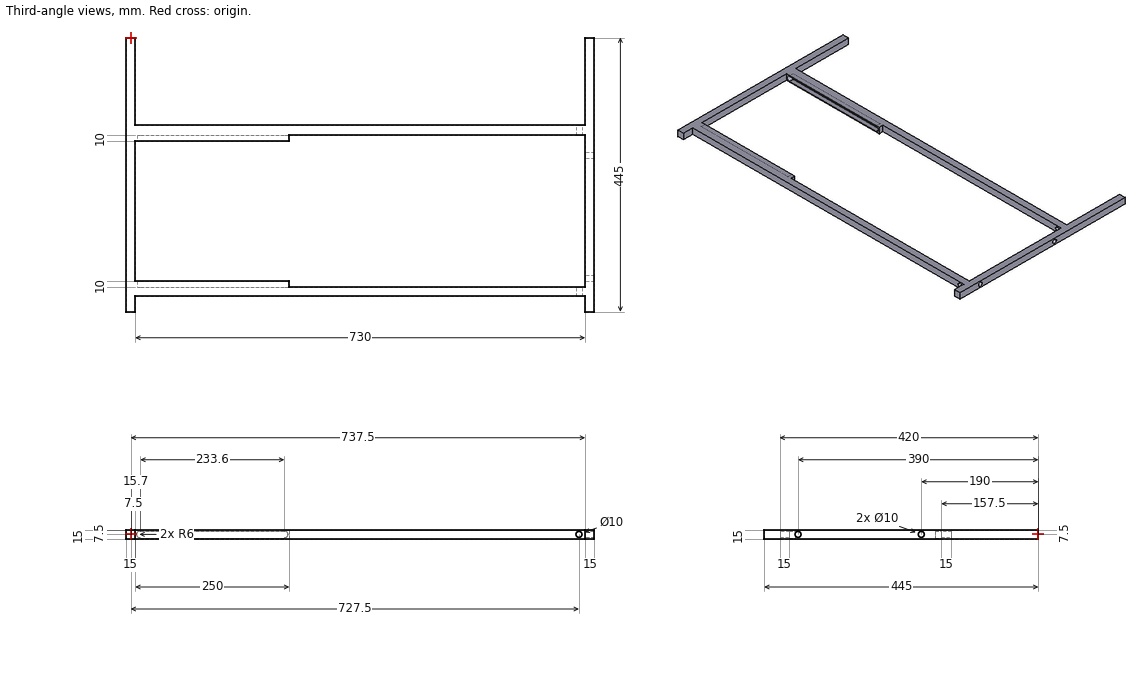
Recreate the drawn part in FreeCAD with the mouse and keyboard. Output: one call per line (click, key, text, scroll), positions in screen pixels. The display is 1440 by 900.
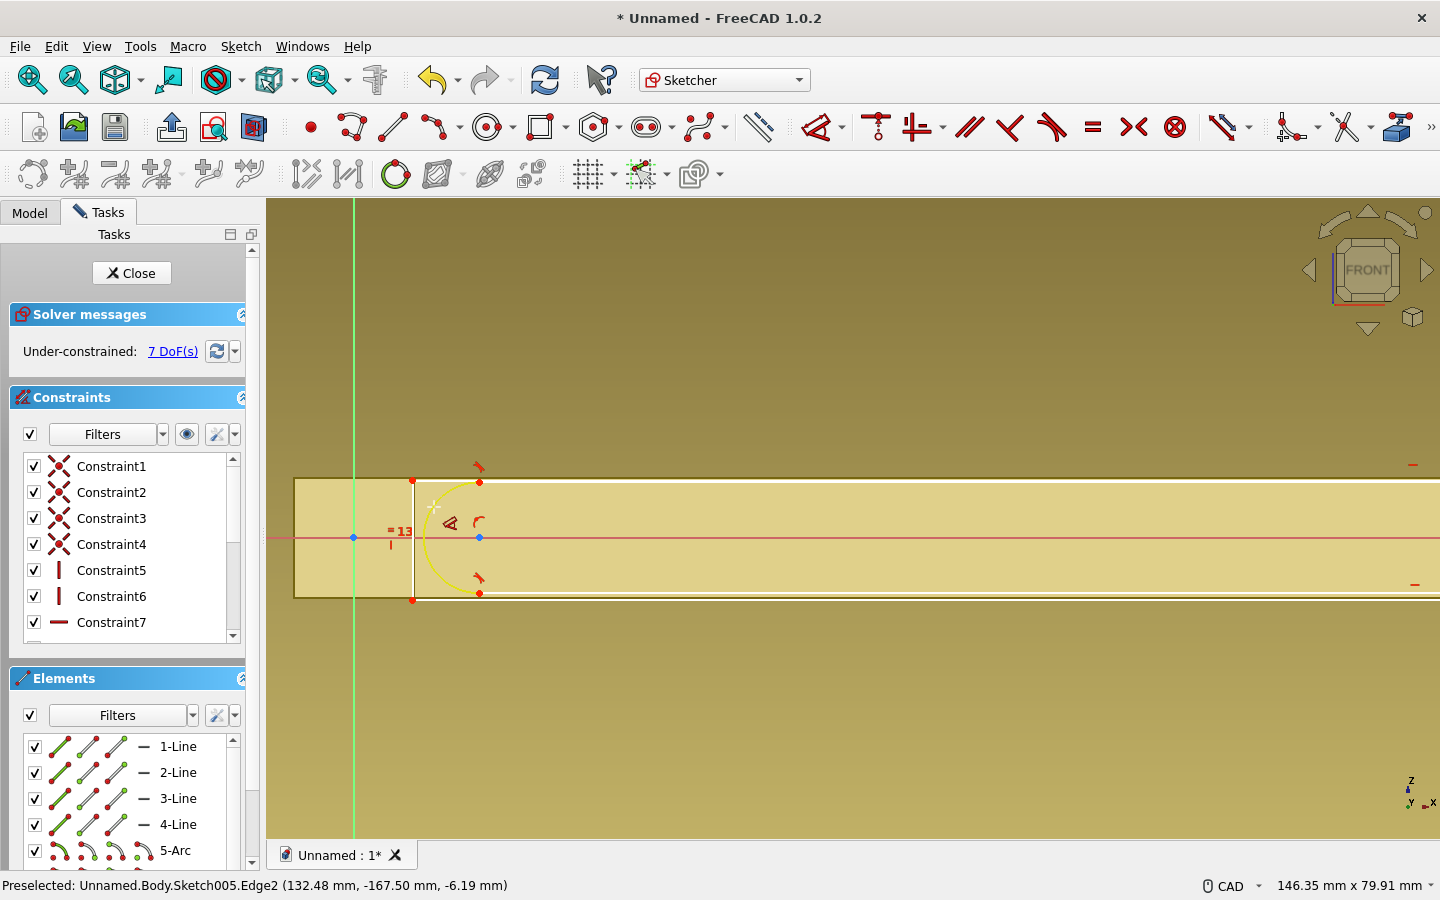
click(434, 505)
click(442, 458)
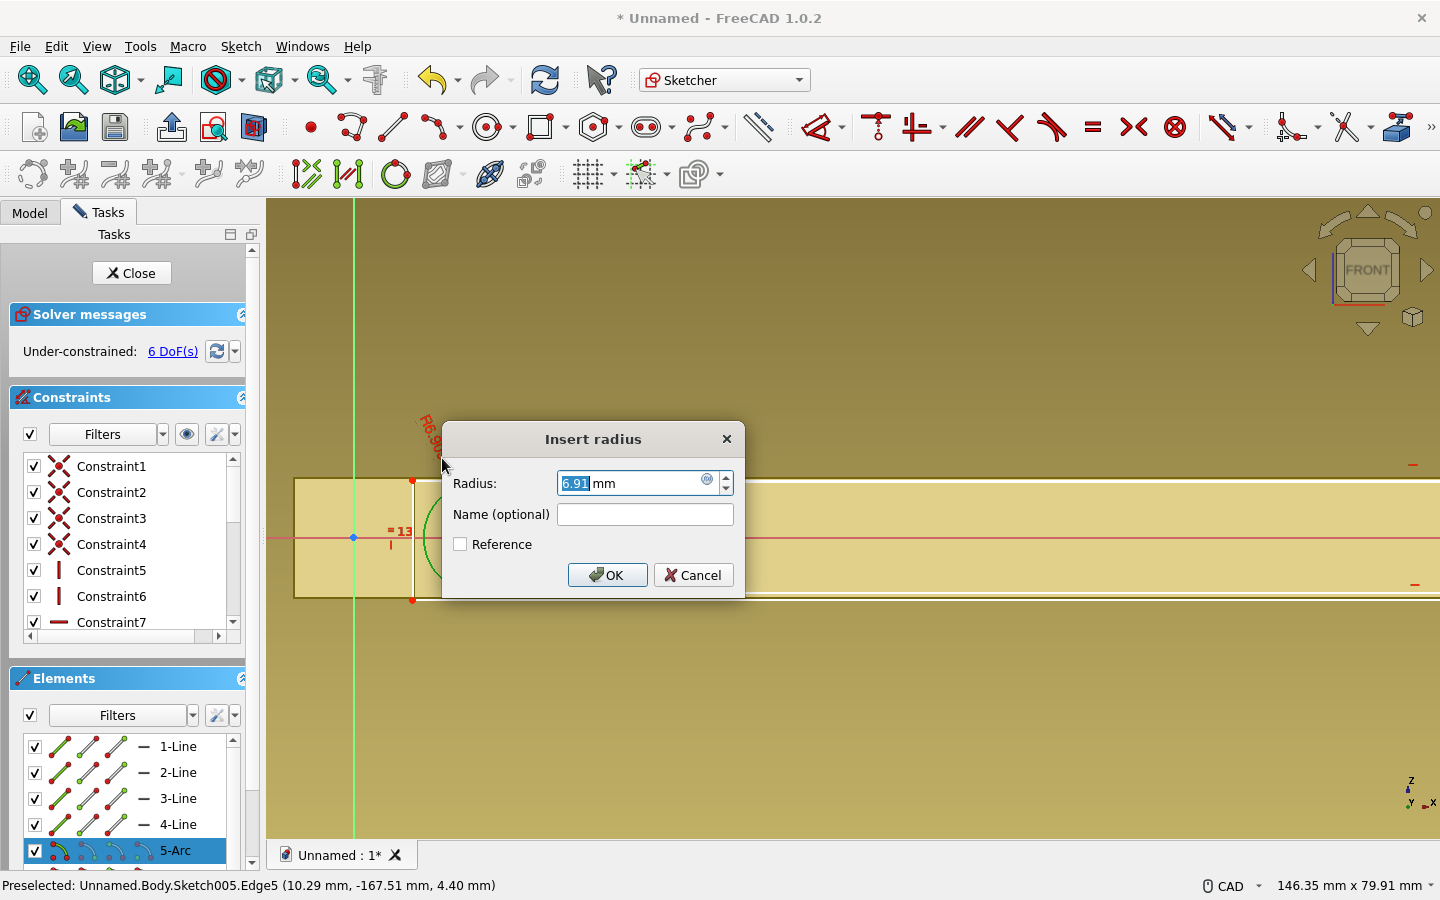
text(6)
key(Return)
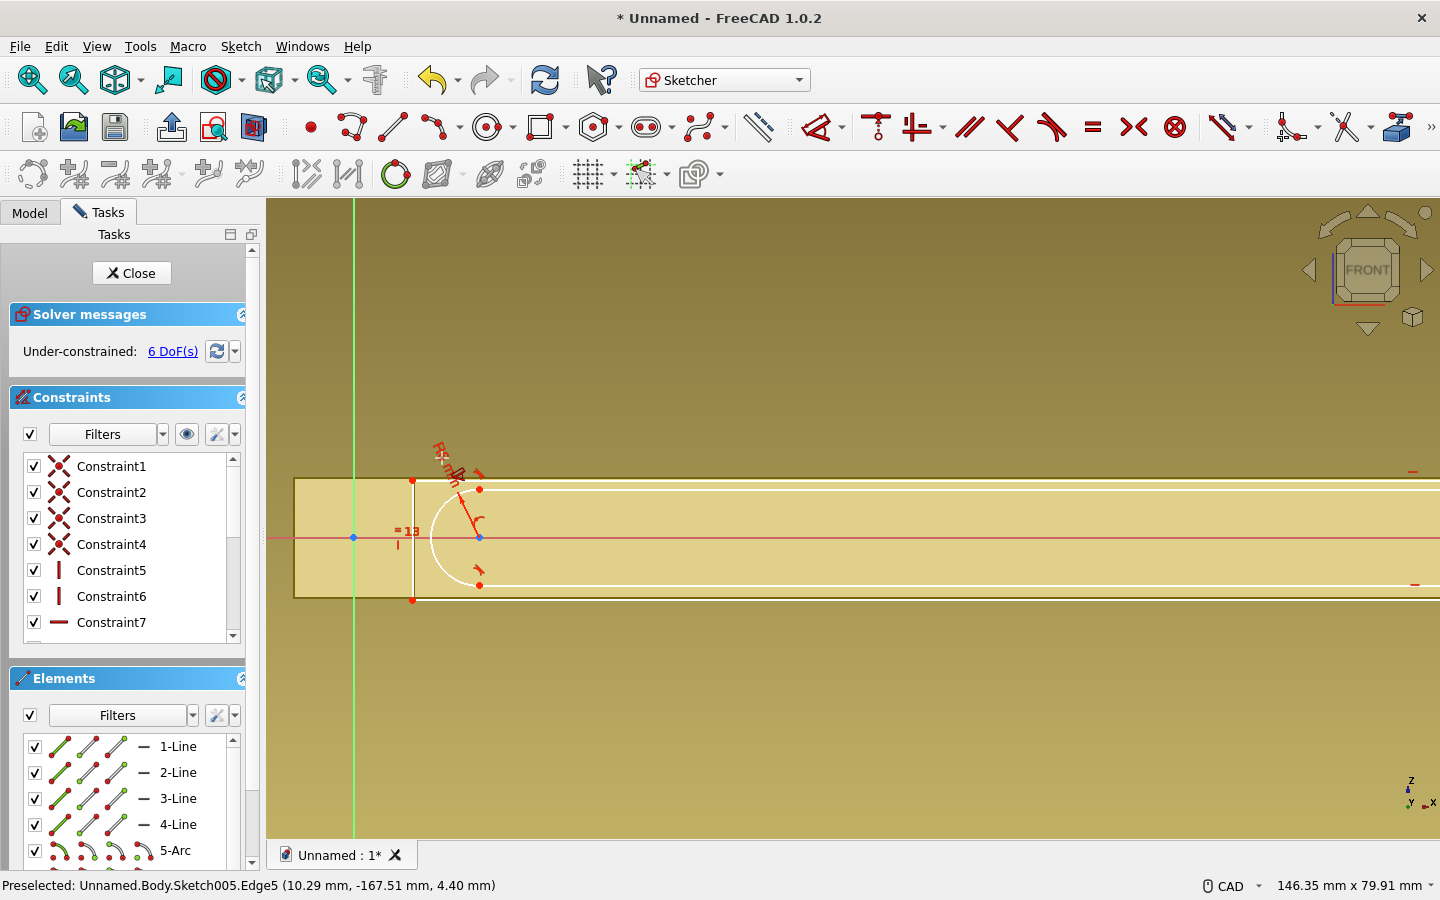
click(413, 517)
click(379, 513)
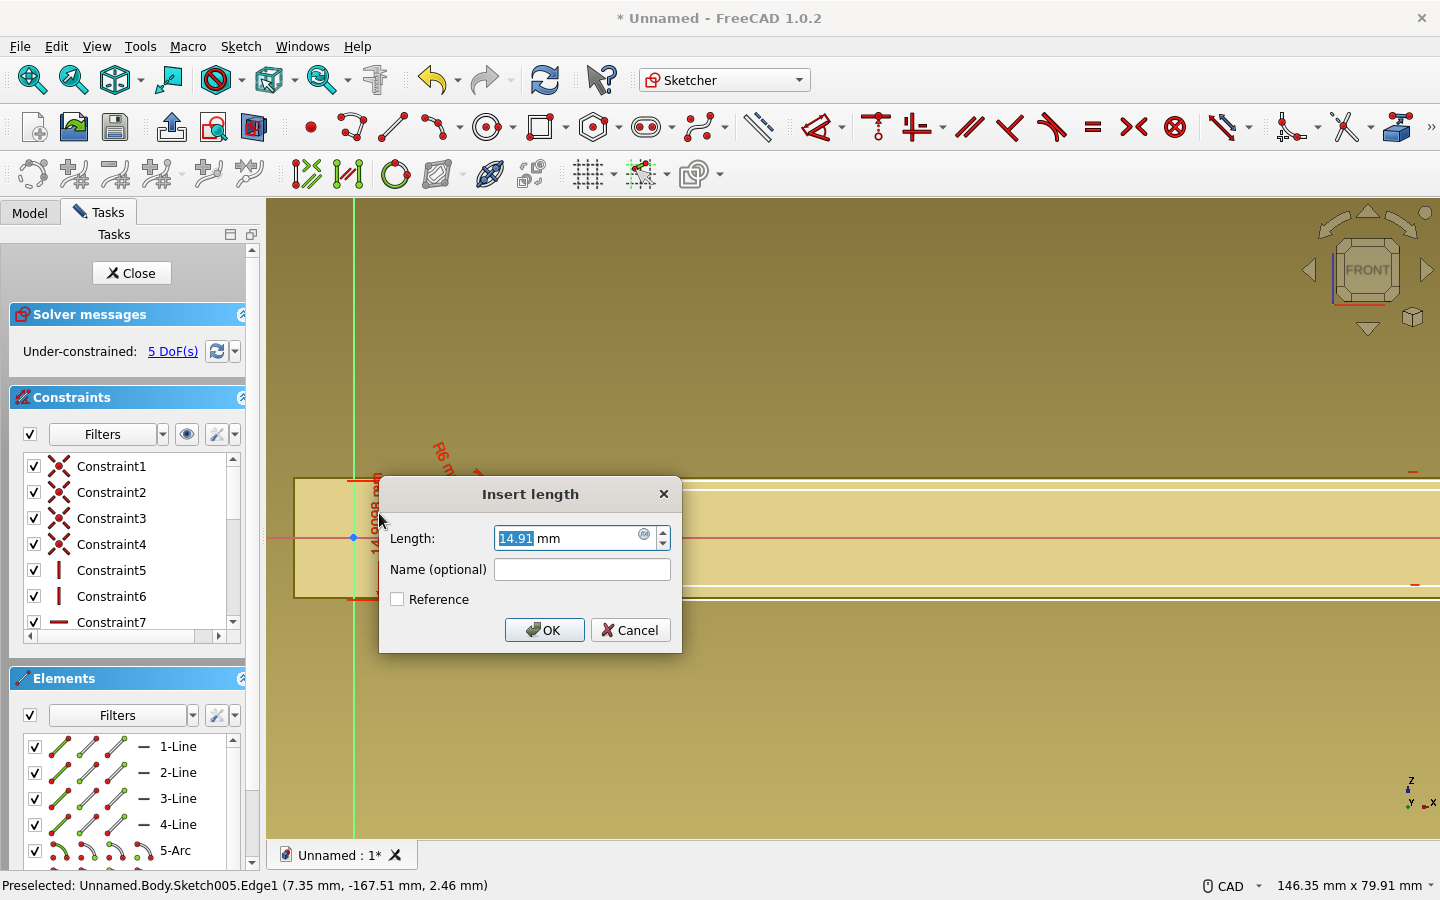
text(15)
key(Return)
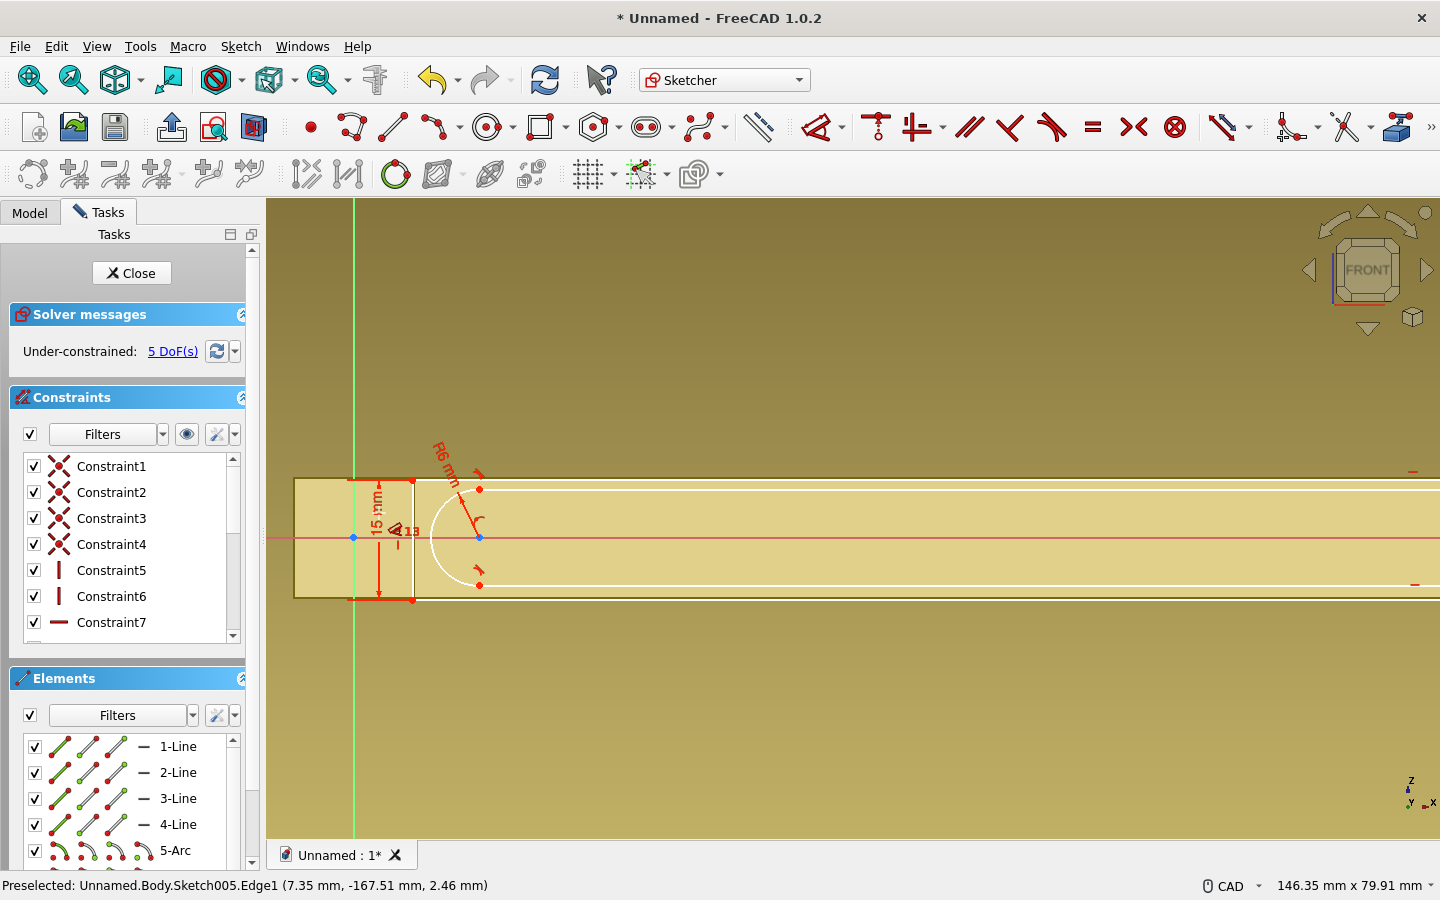
click(1015, 600)
click(844, 634)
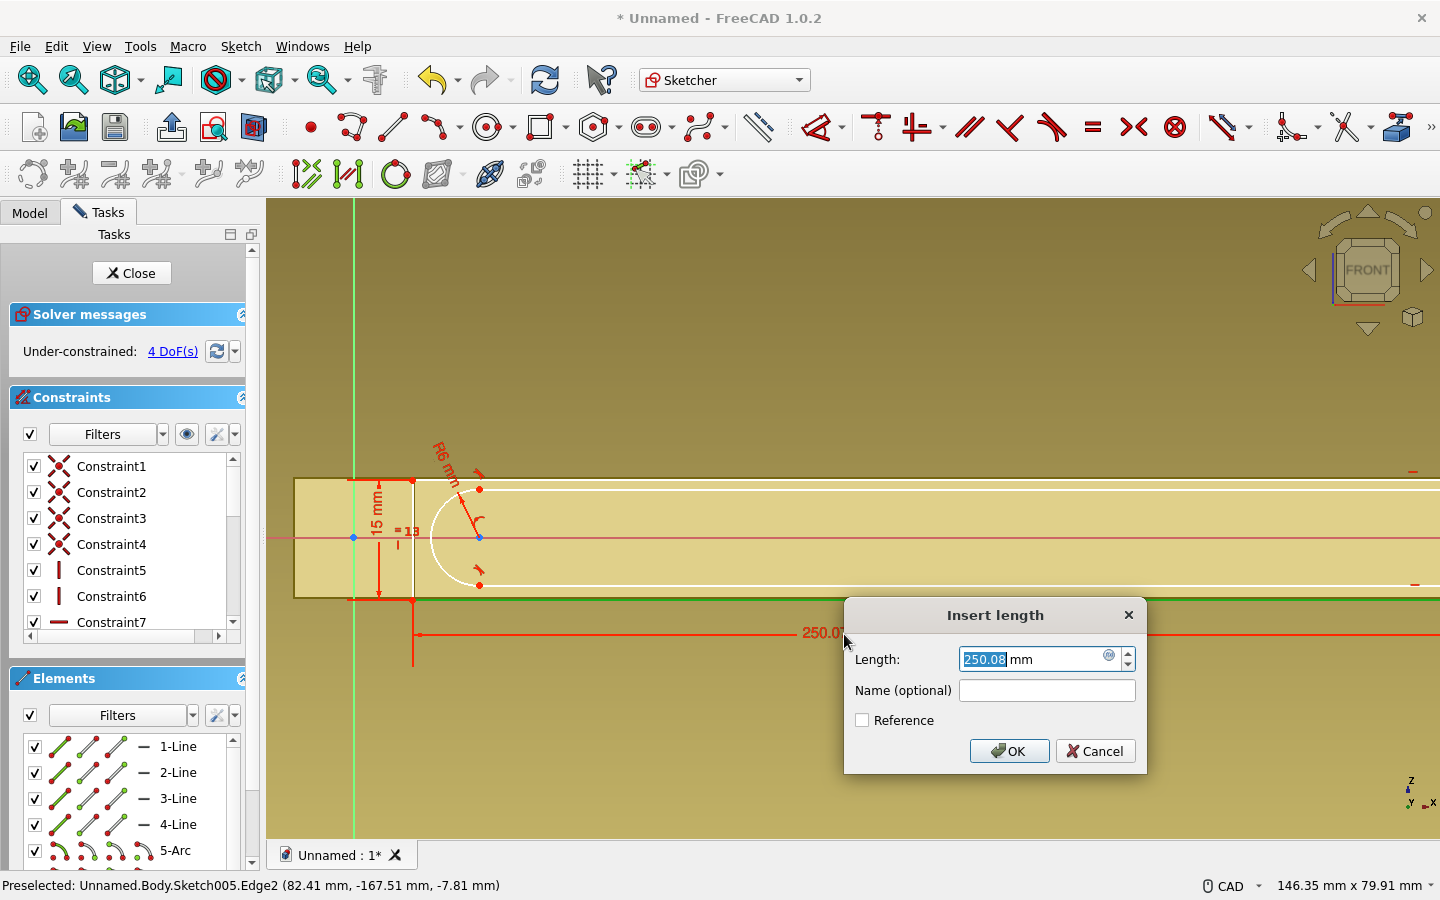
text(250)
key(Return)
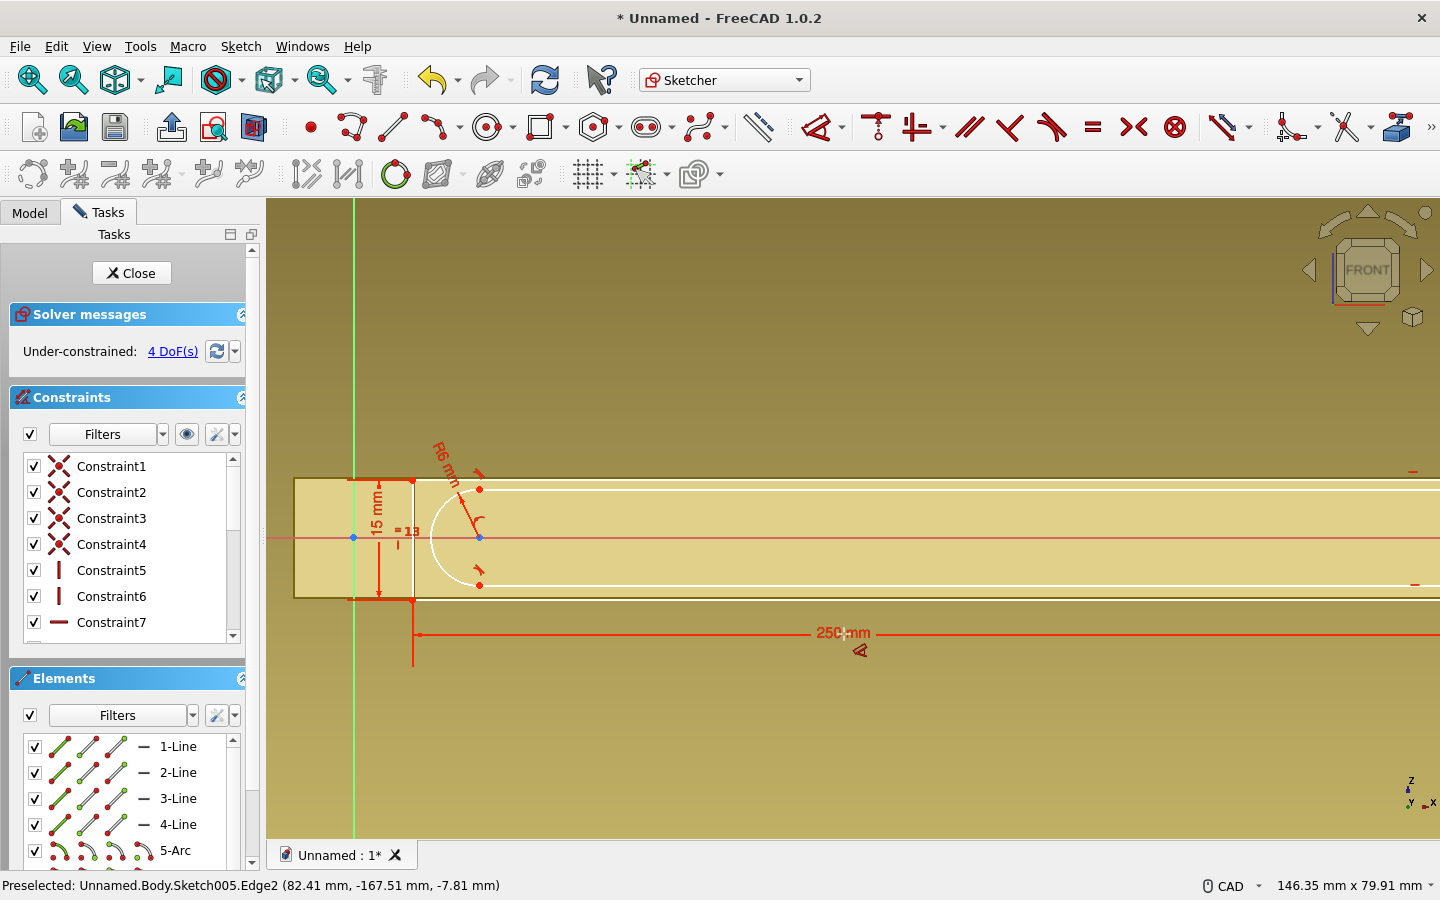
click(413, 480)
click(370, 446)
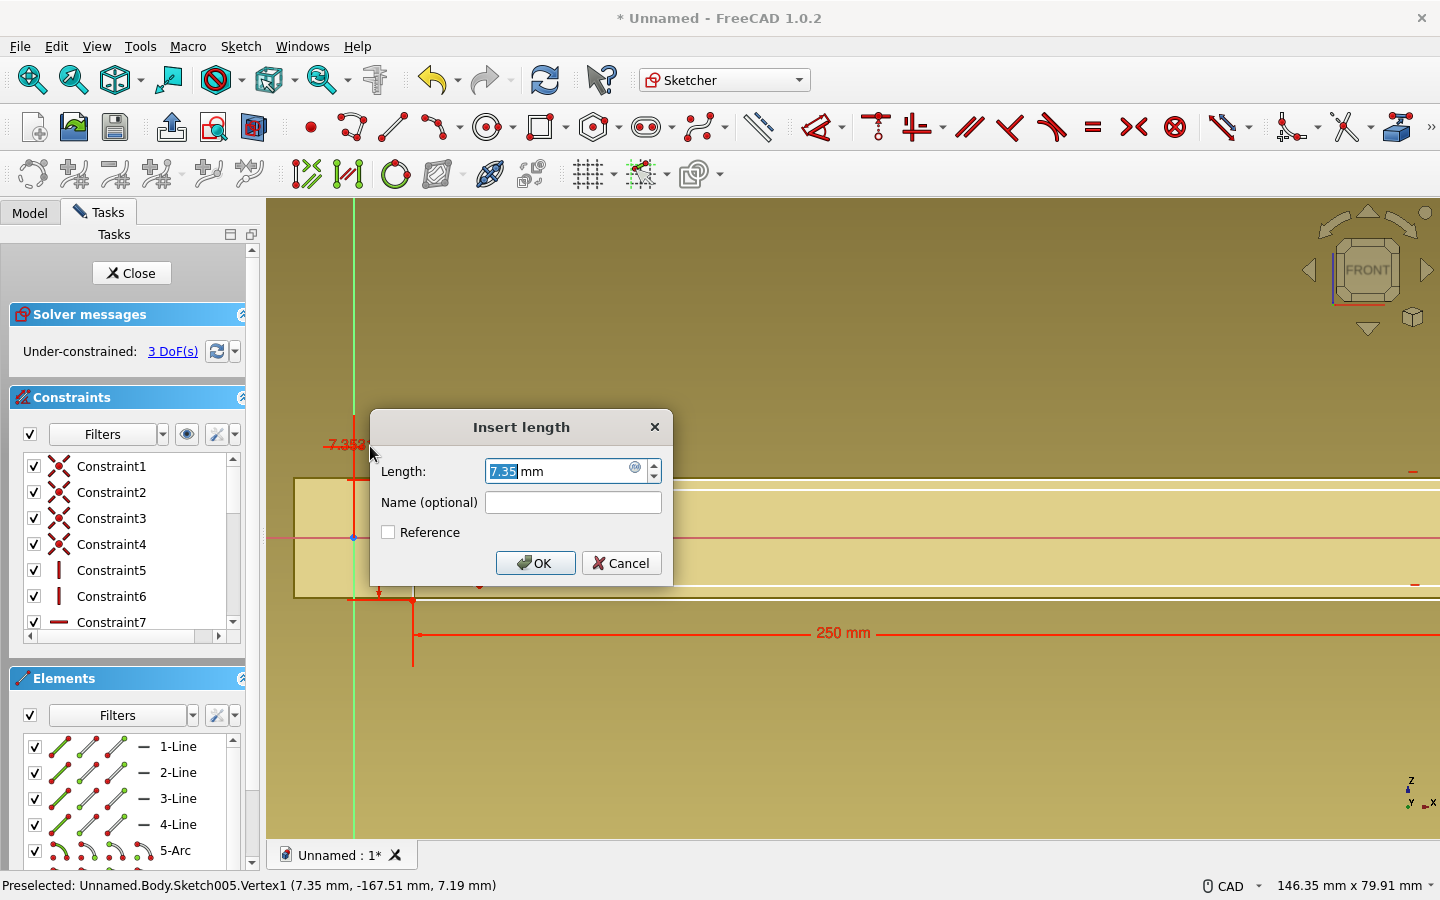
text(7.5)
key(Return)